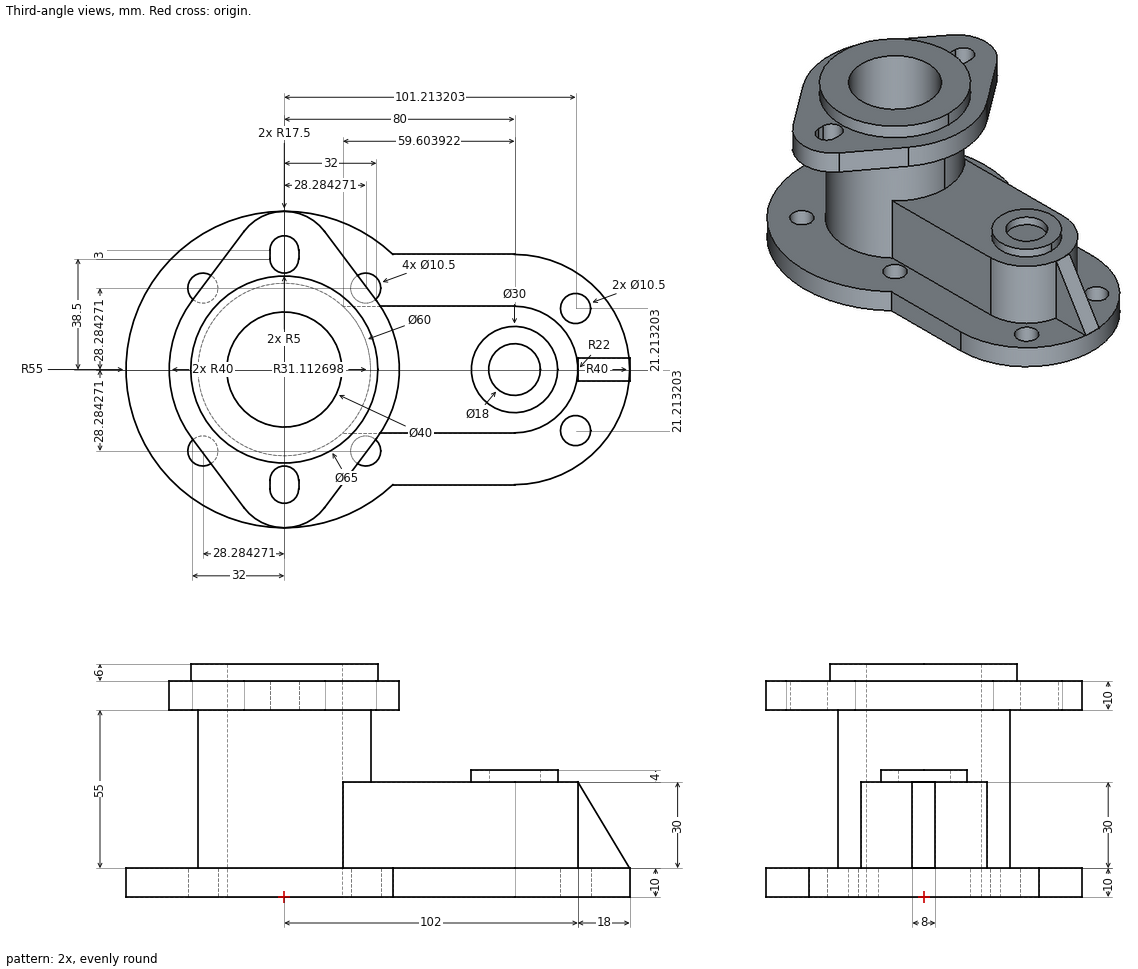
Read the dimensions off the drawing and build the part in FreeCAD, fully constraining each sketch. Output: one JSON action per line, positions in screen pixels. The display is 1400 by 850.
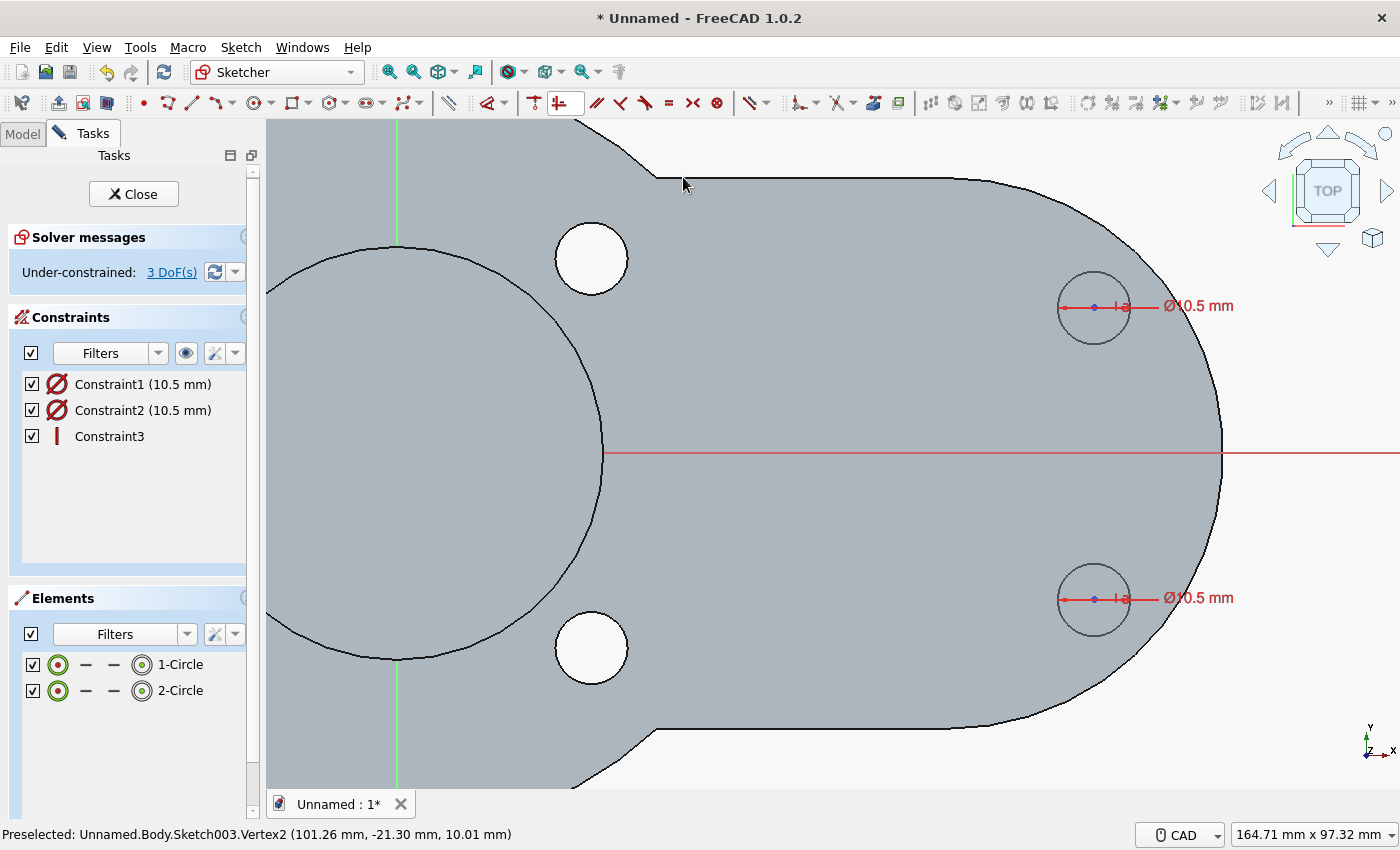
{"action": "key", "text": "d"}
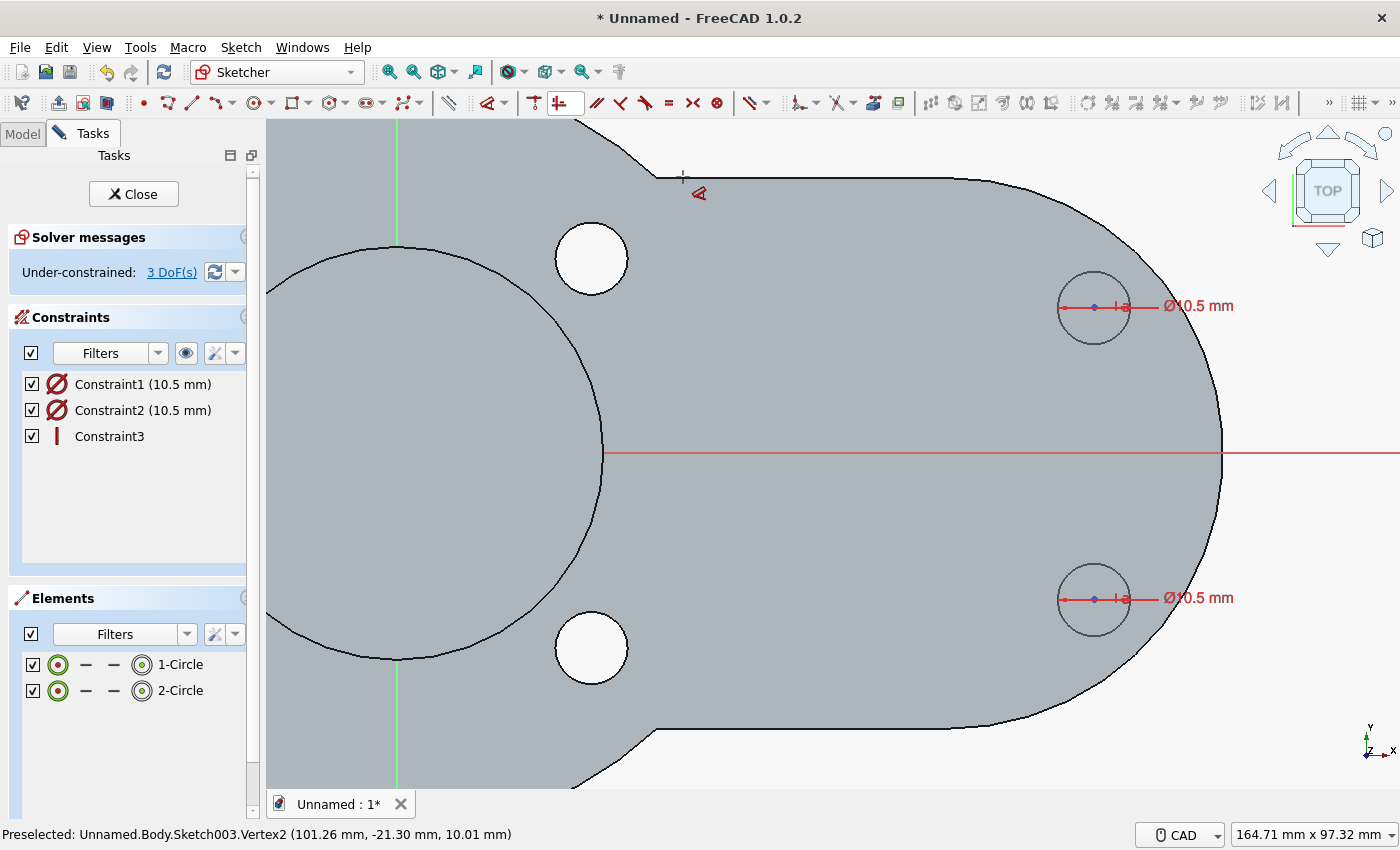
{"action": "left_click", "coordinate": [1094, 308]}
{"action": "left_click", "coordinate": [363, 381]}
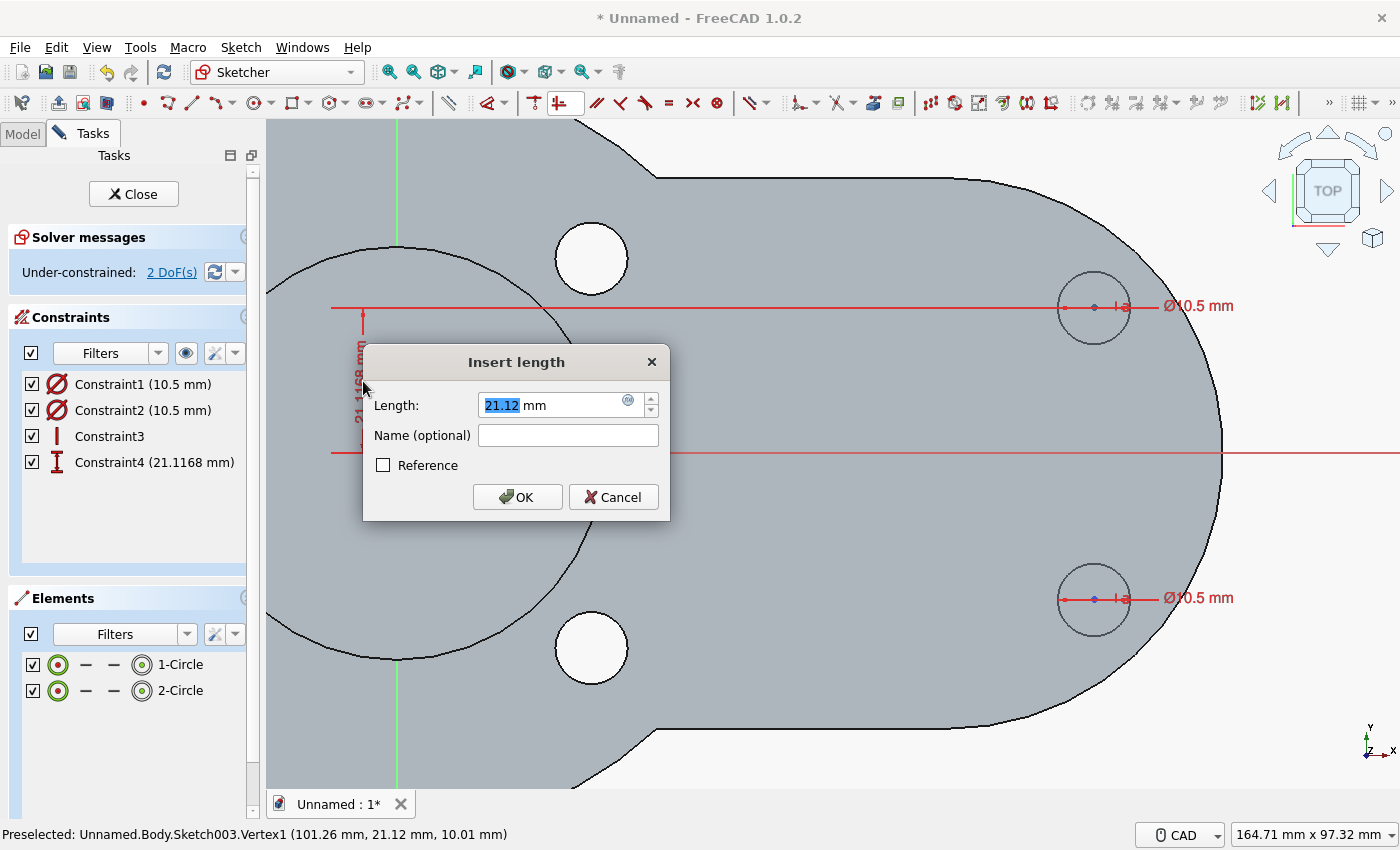
{"action": "type", "text": "21.213203"}
{"action": "key", "text": "Return"}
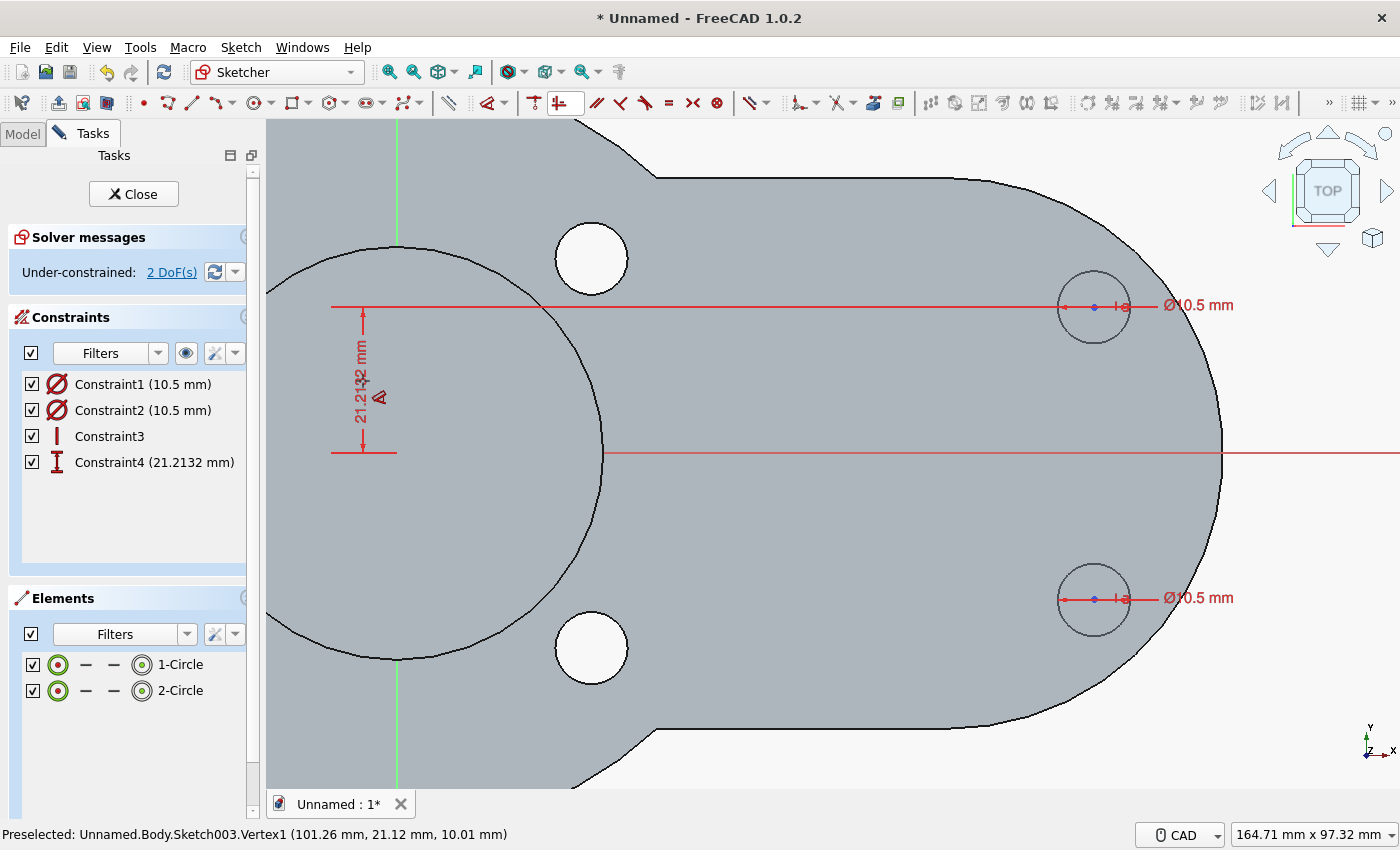
{"action": "left_click", "coordinate": [1094, 600]}
{"action": "left_click", "coordinate": [363, 527]}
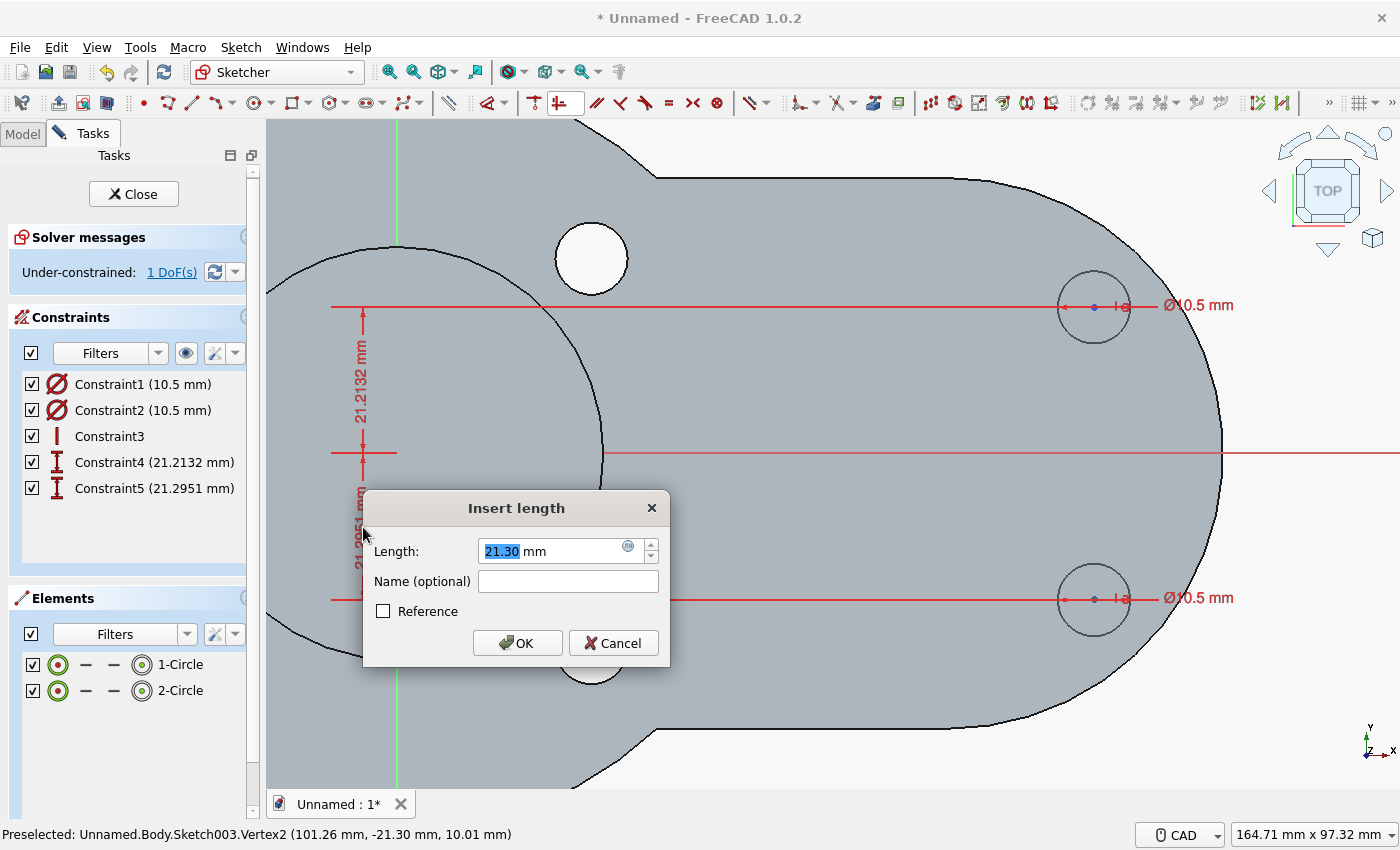
{"action": "type", "text": "21.213203"}
{"action": "key", "text": "Return"}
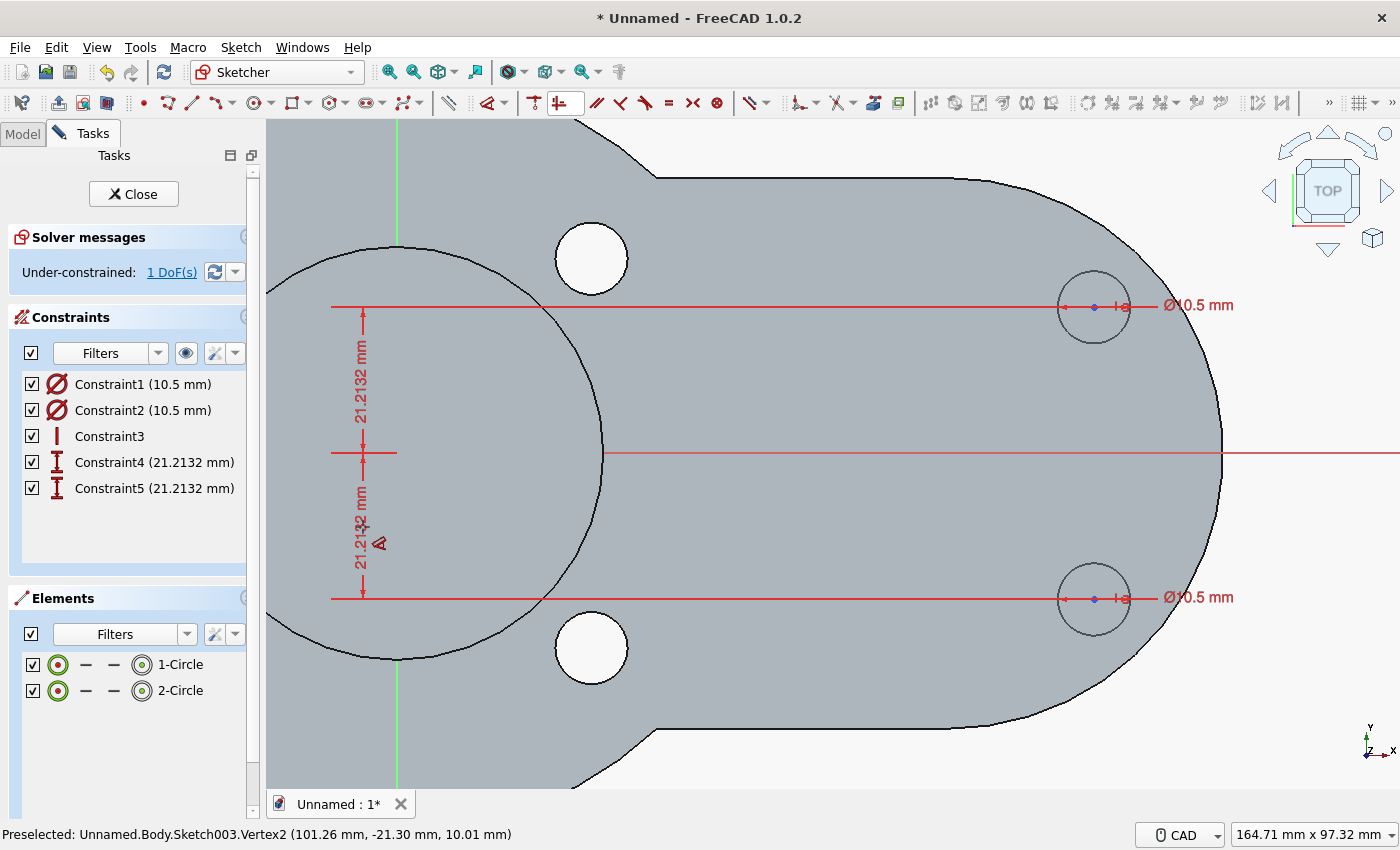
{"action": "left_click", "coordinate": [1094, 307]}
{"action": "left_click", "coordinate": [745, 273]}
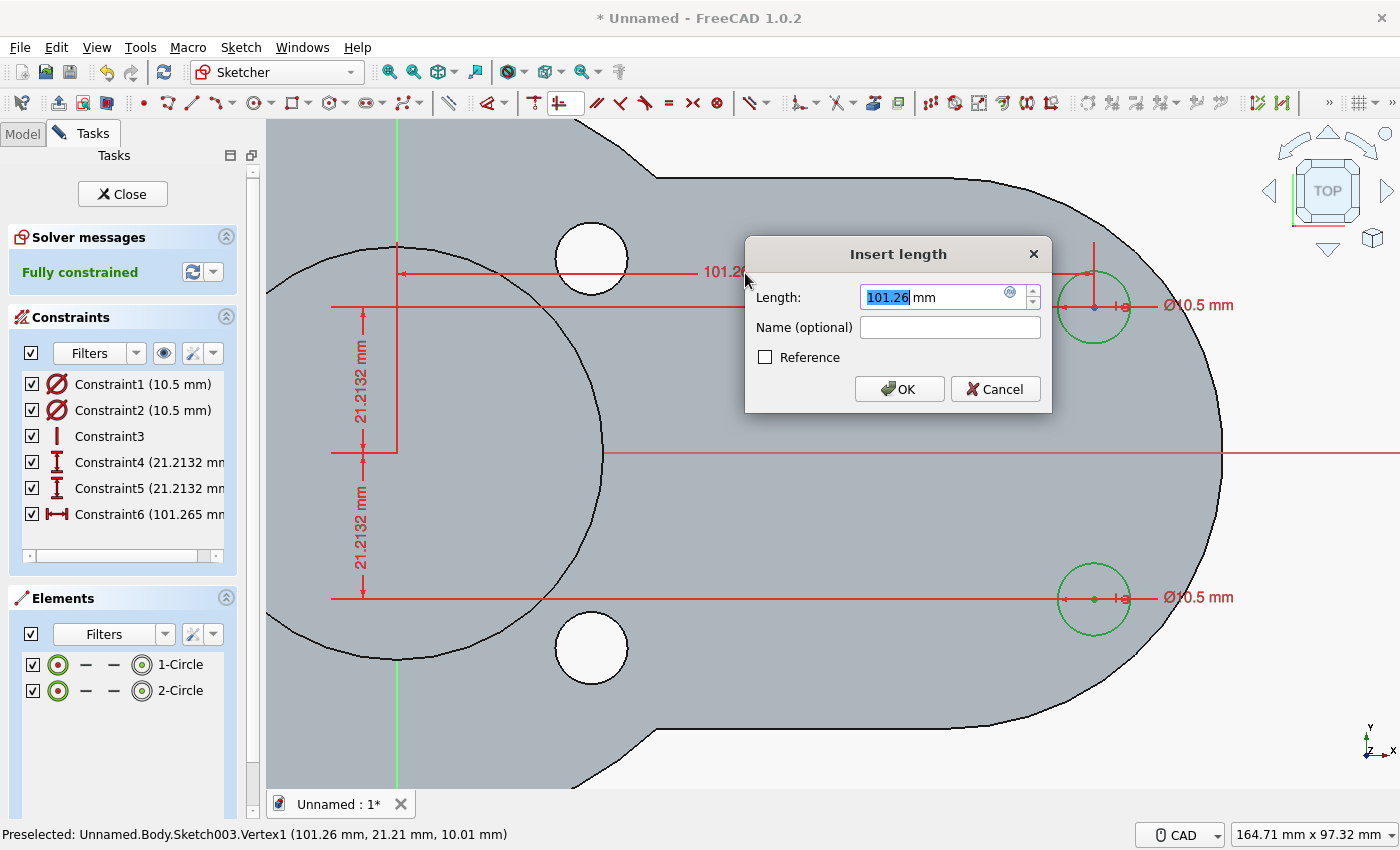
{"action": "type", "text": "101.213203"}
{"action": "key", "text": "Return"}
{"action": "key", "text": "Escape"}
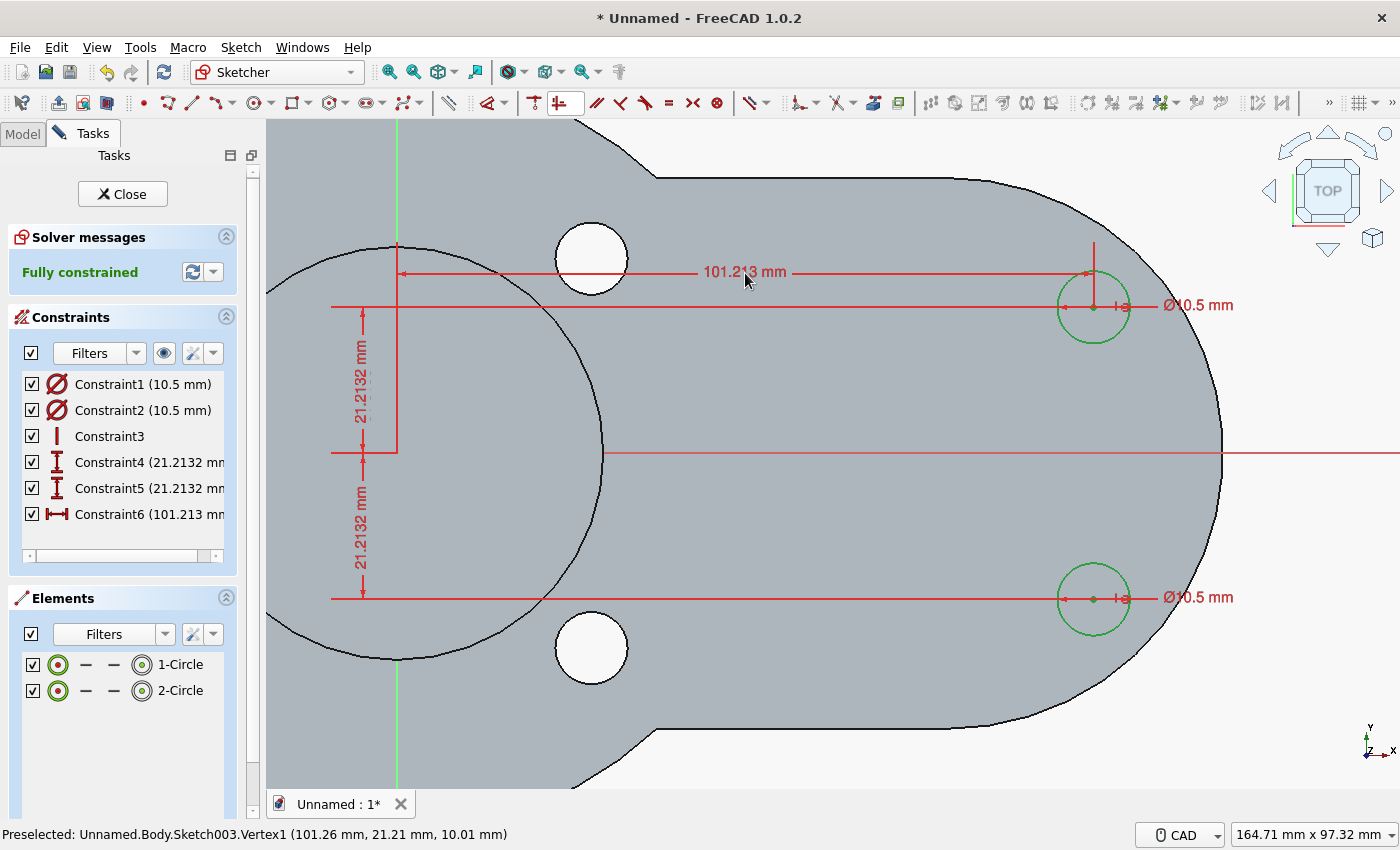
{"action": "left_click", "coordinate": [123, 194]}